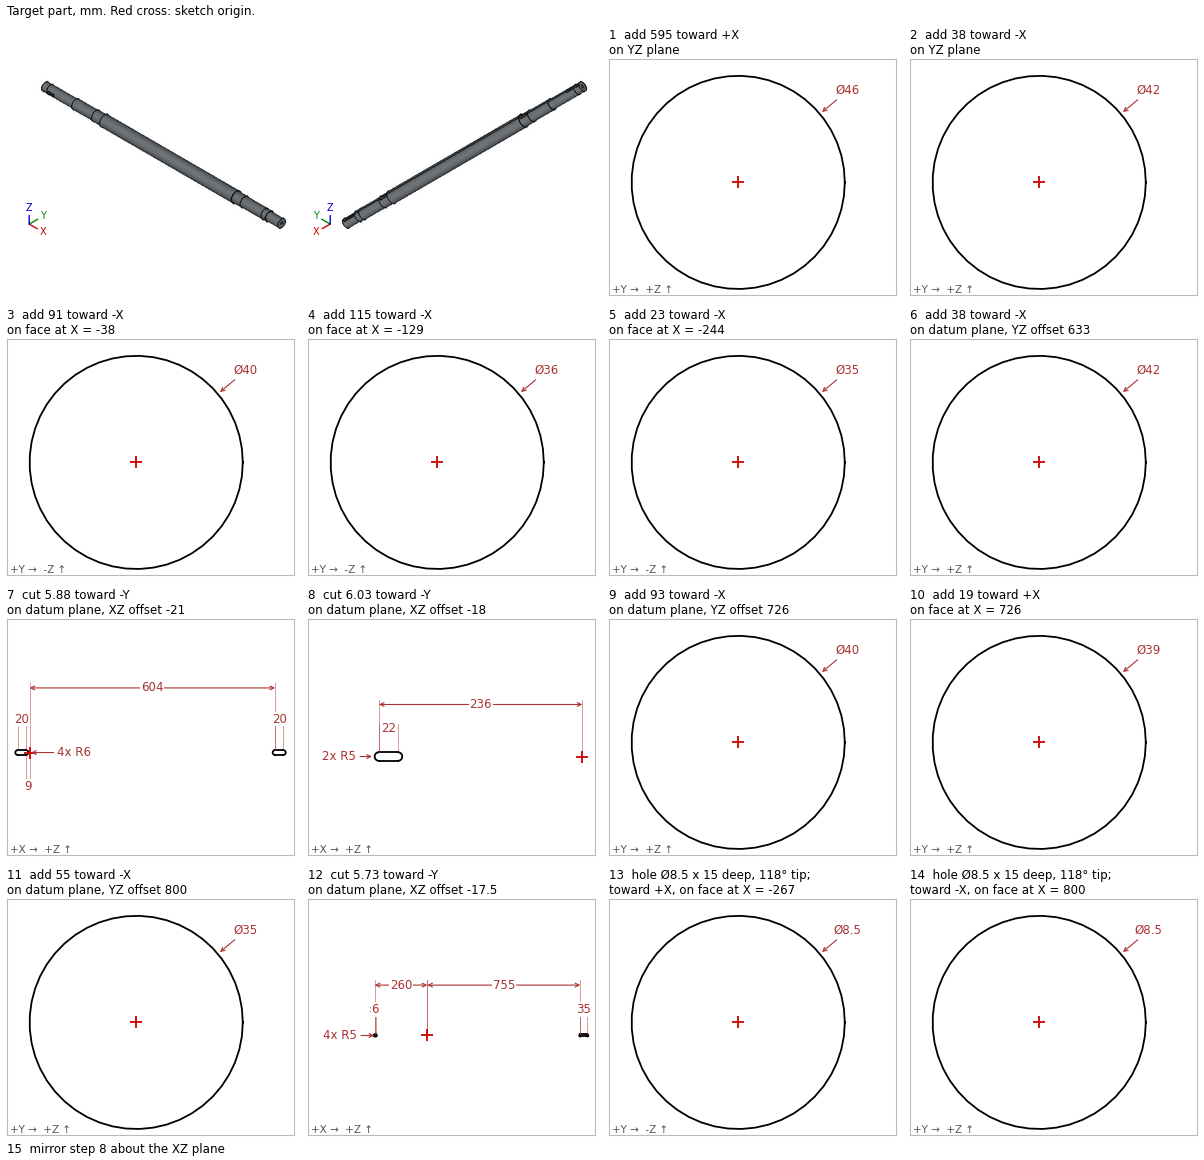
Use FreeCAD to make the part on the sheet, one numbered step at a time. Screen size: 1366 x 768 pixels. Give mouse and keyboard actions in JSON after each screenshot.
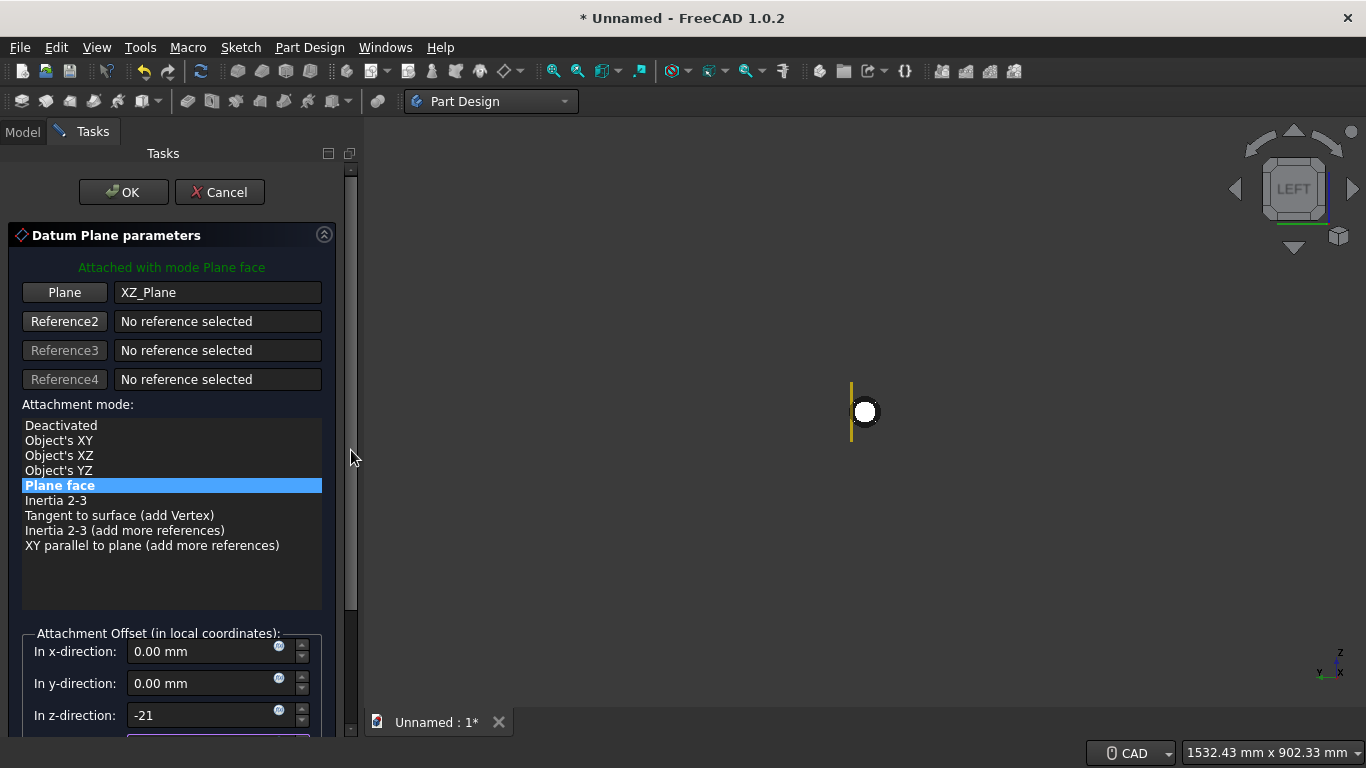
{"action": "left_click", "coordinate": [124, 192]}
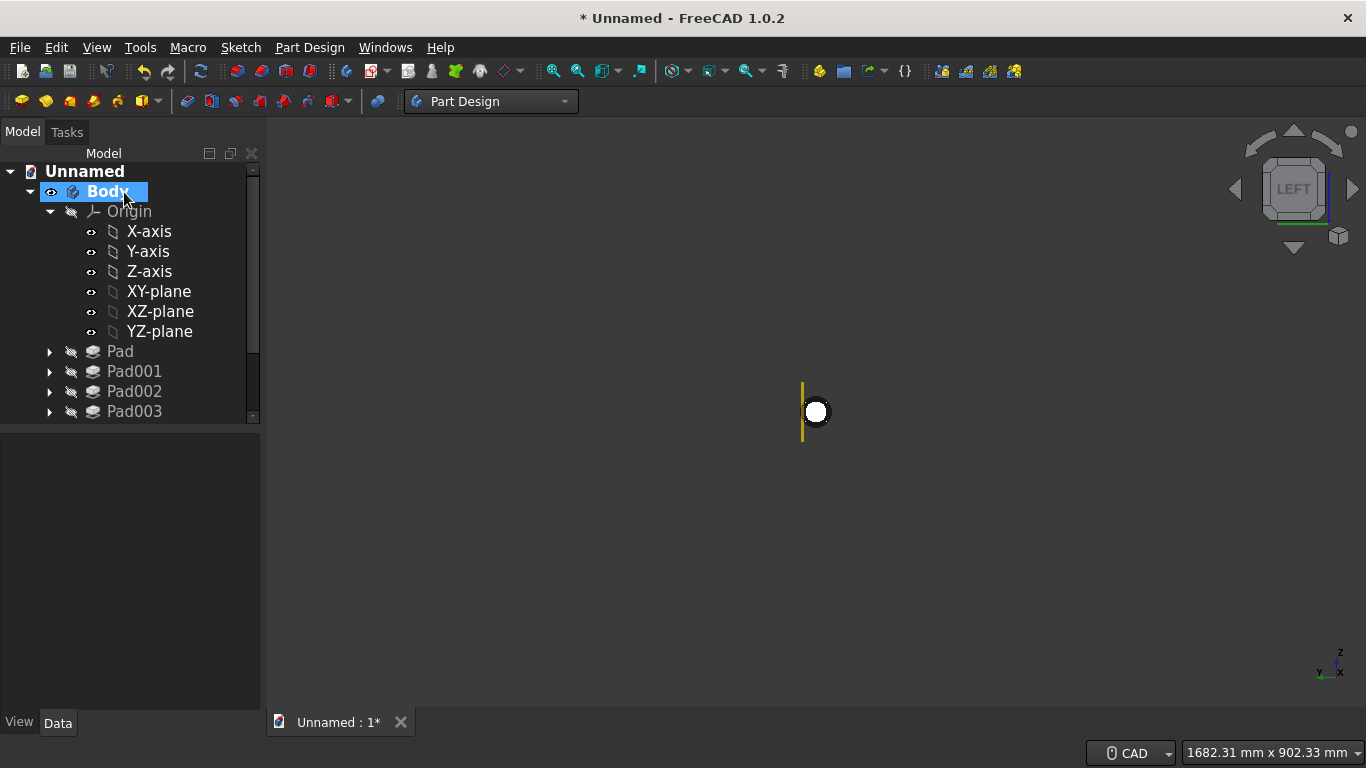
{"action": "scroll", "coordinate": [100, 287], "scroll_direction": "down", "scroll_amount": 3}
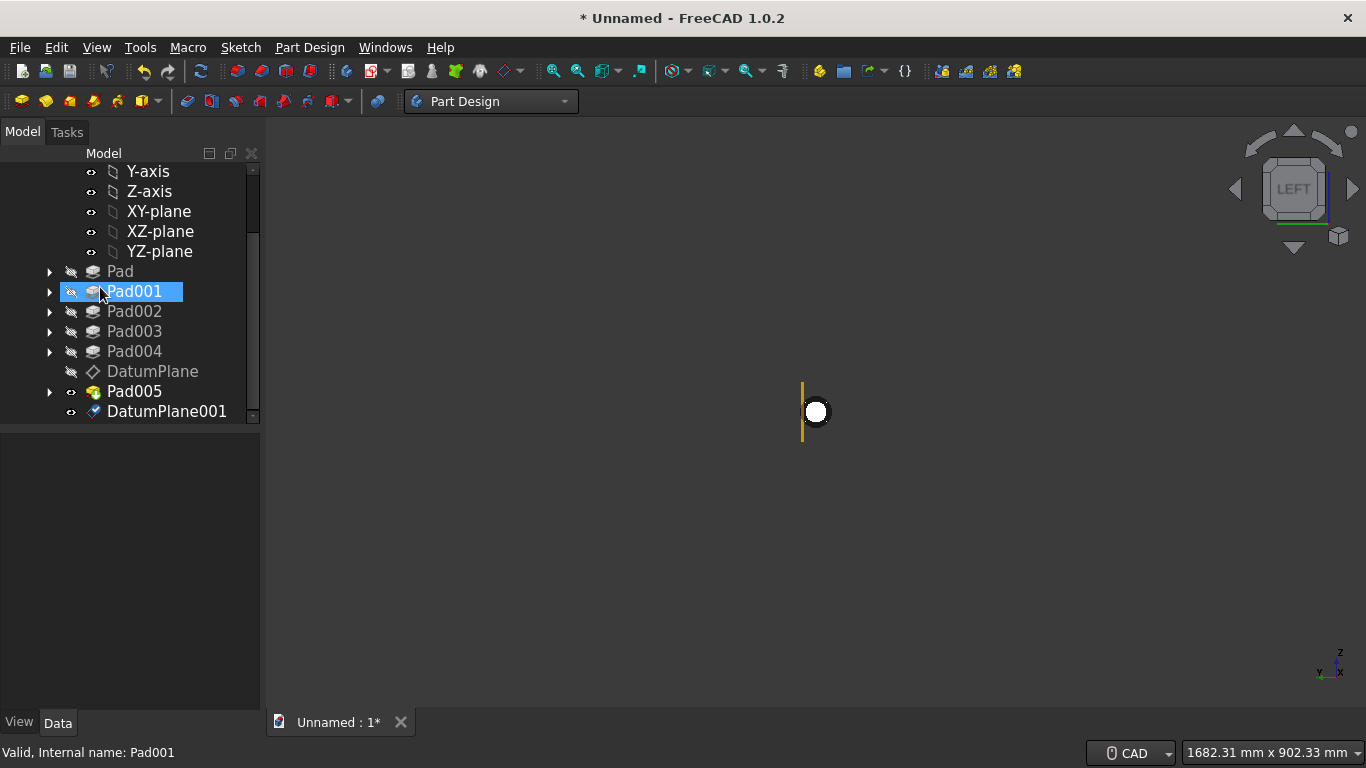
{"action": "left_click", "coordinate": [116, 412]}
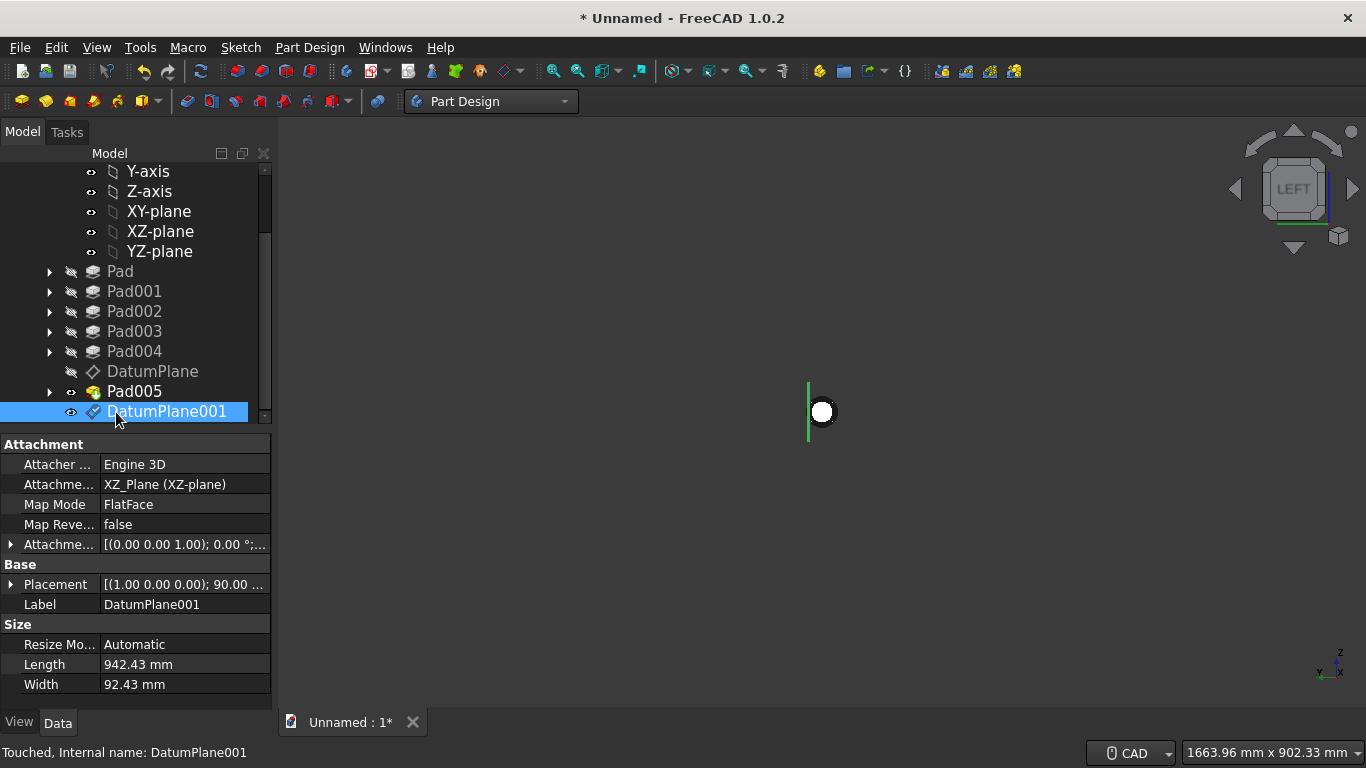
{"action": "left_click", "coordinate": [372, 72]}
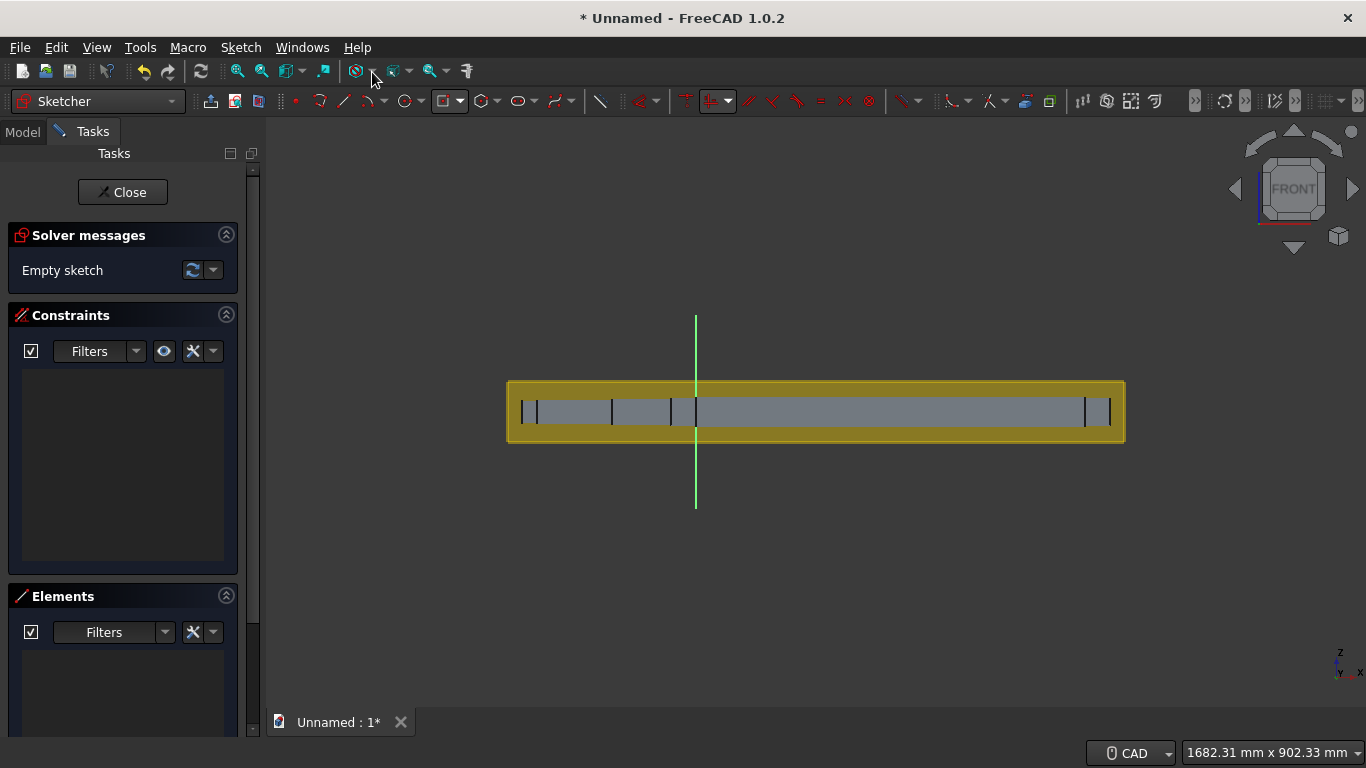
{"action": "left_click", "coordinate": [260, 102]}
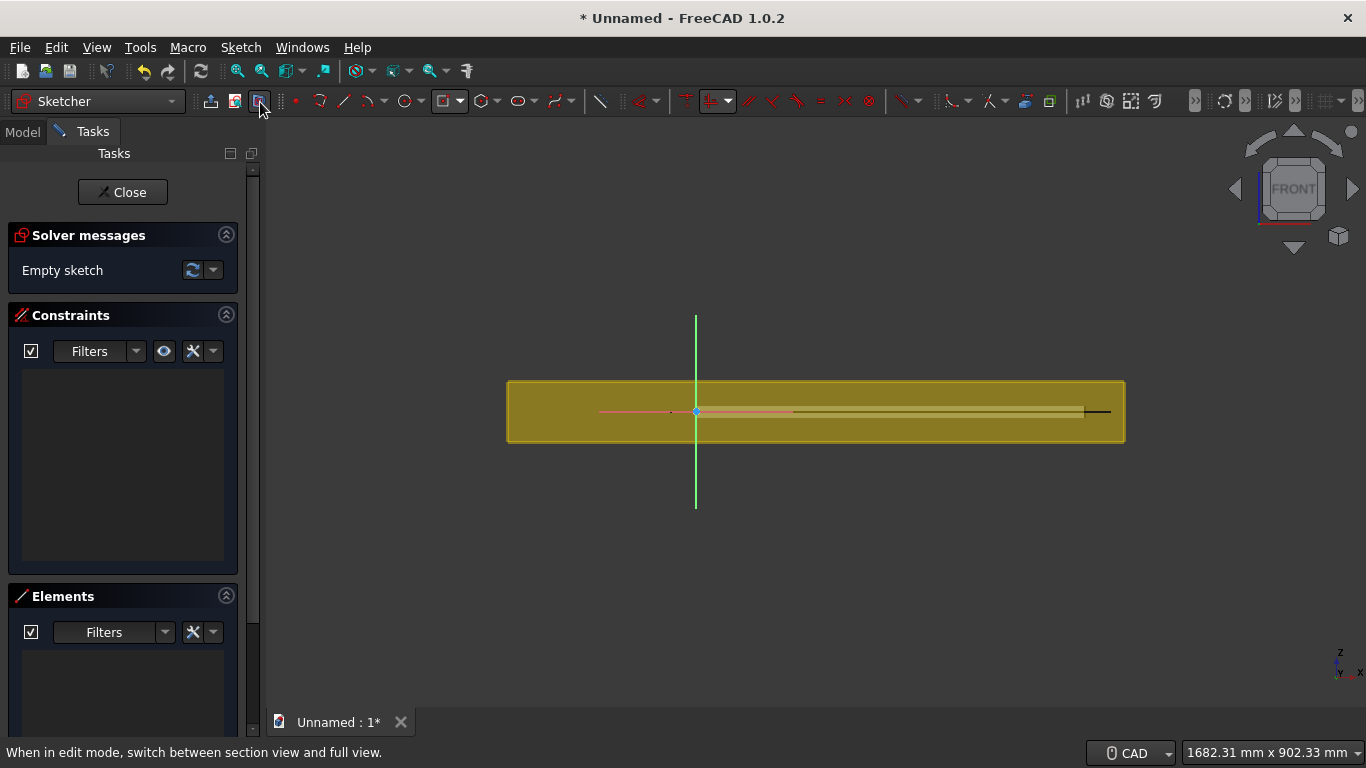
{"action": "scroll", "coordinate": [1182, 412], "scroll_direction": "up", "scroll_amount": 2}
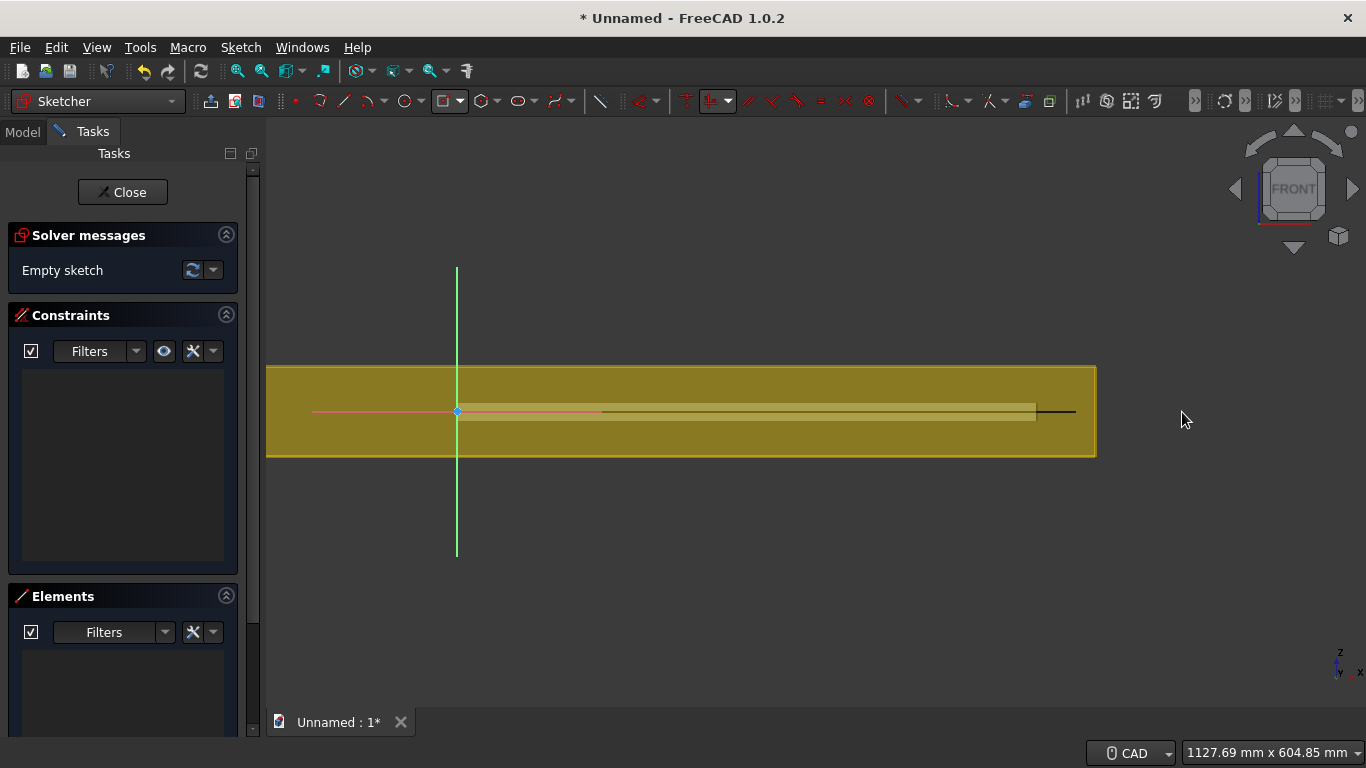
{"action": "key", "text": "g s"}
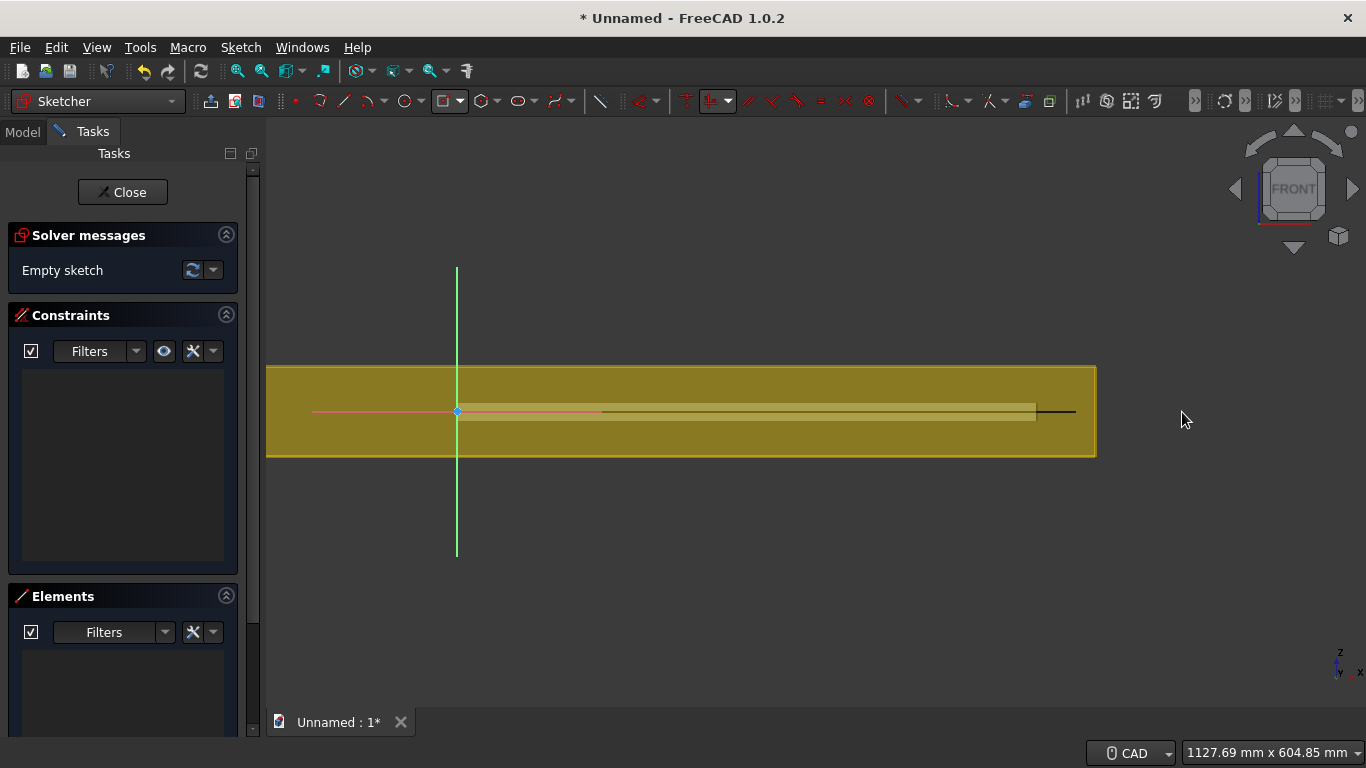
{"action": "scroll", "coordinate": [429, 412], "scroll_direction": "up", "scroll_amount": 7}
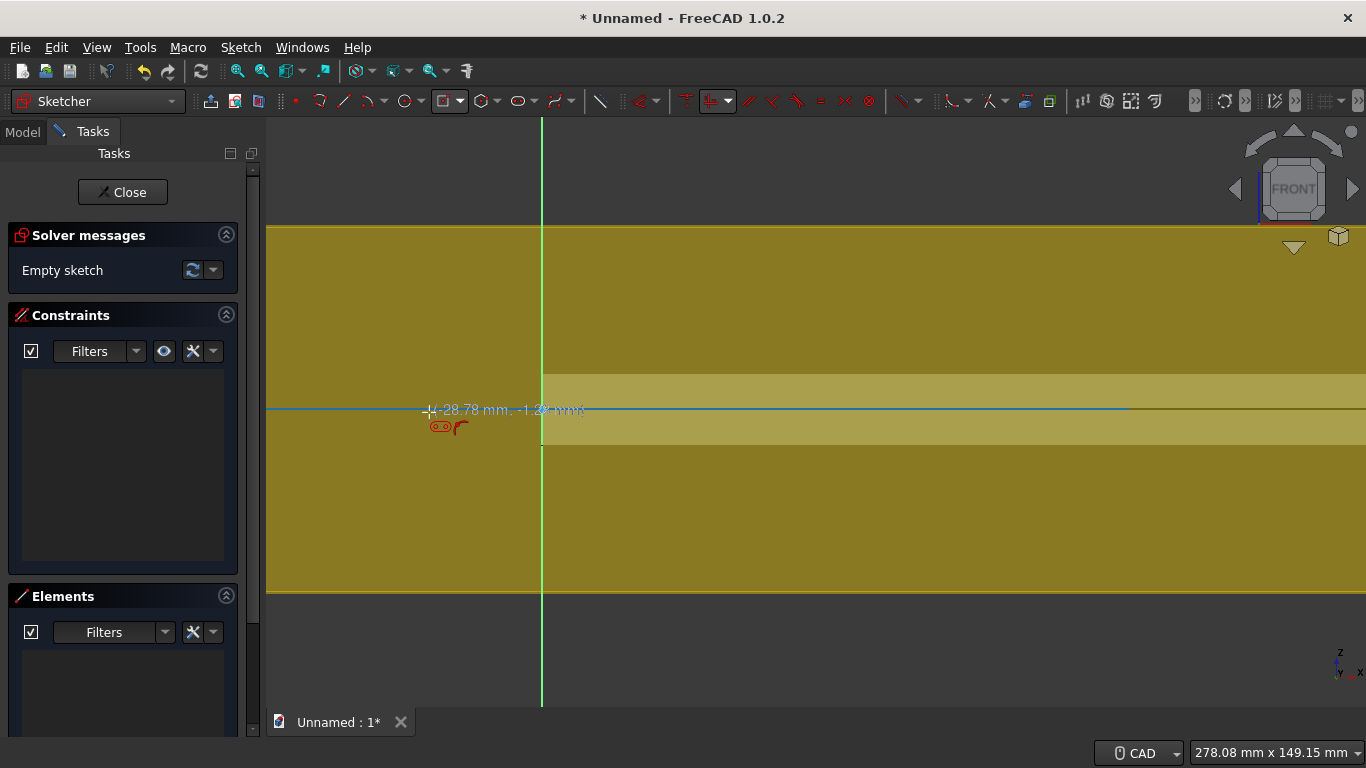
{"action": "scroll", "coordinate": [429, 413], "scroll_direction": "down", "scroll_amount": 7}